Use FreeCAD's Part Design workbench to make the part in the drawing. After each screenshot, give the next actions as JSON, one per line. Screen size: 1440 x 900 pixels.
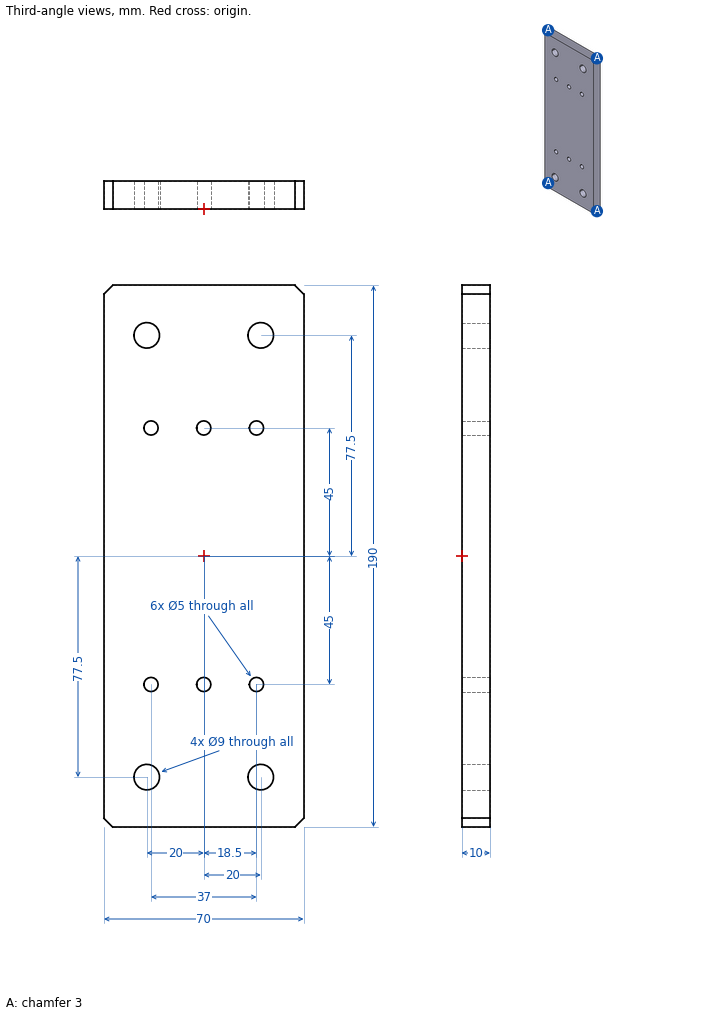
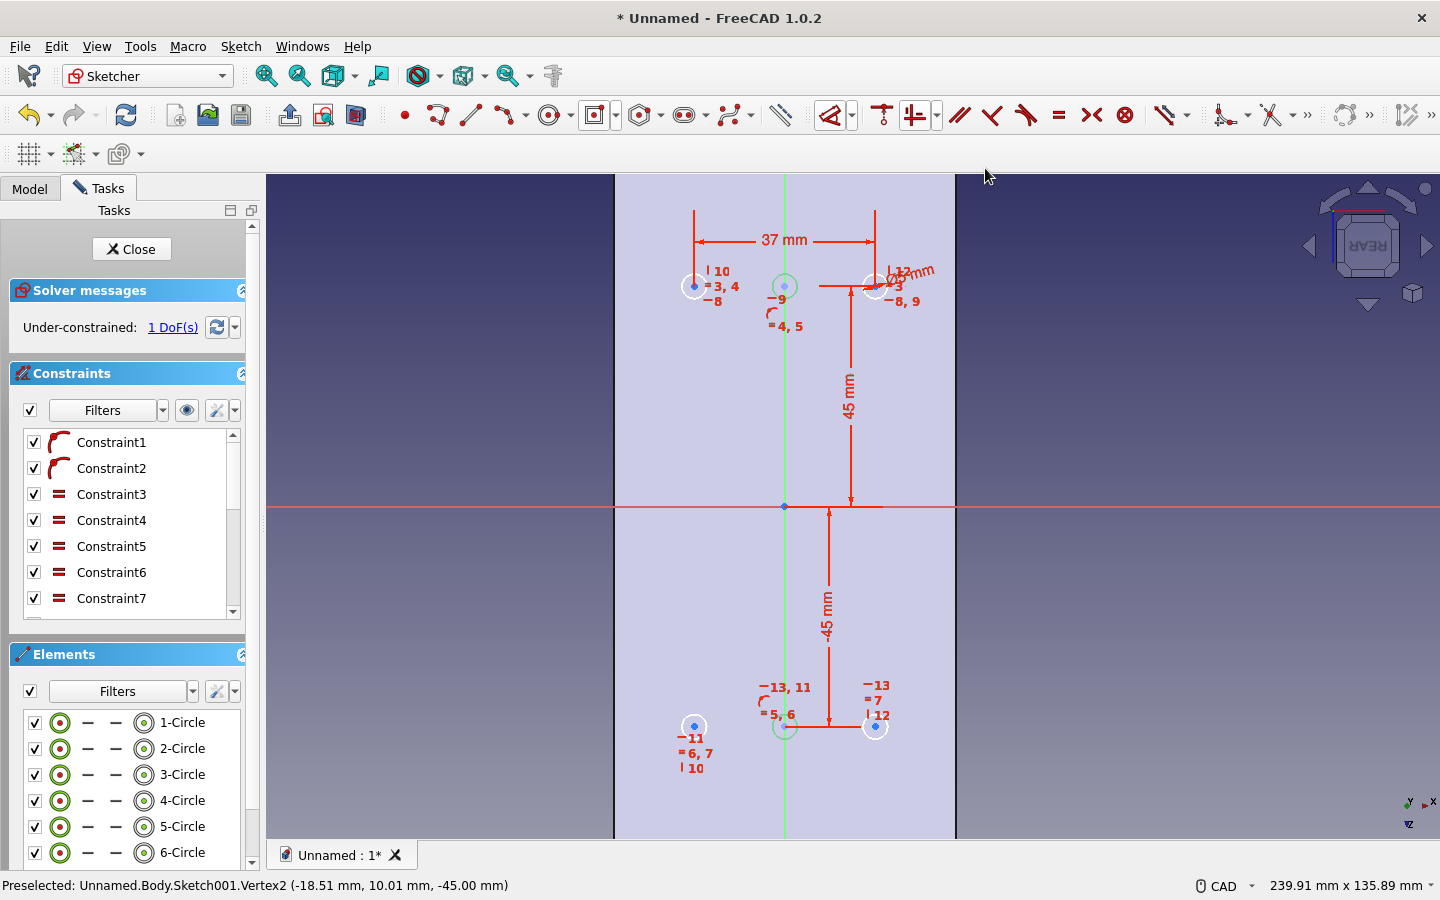
{"action": "left_click", "coordinate": [875, 286]}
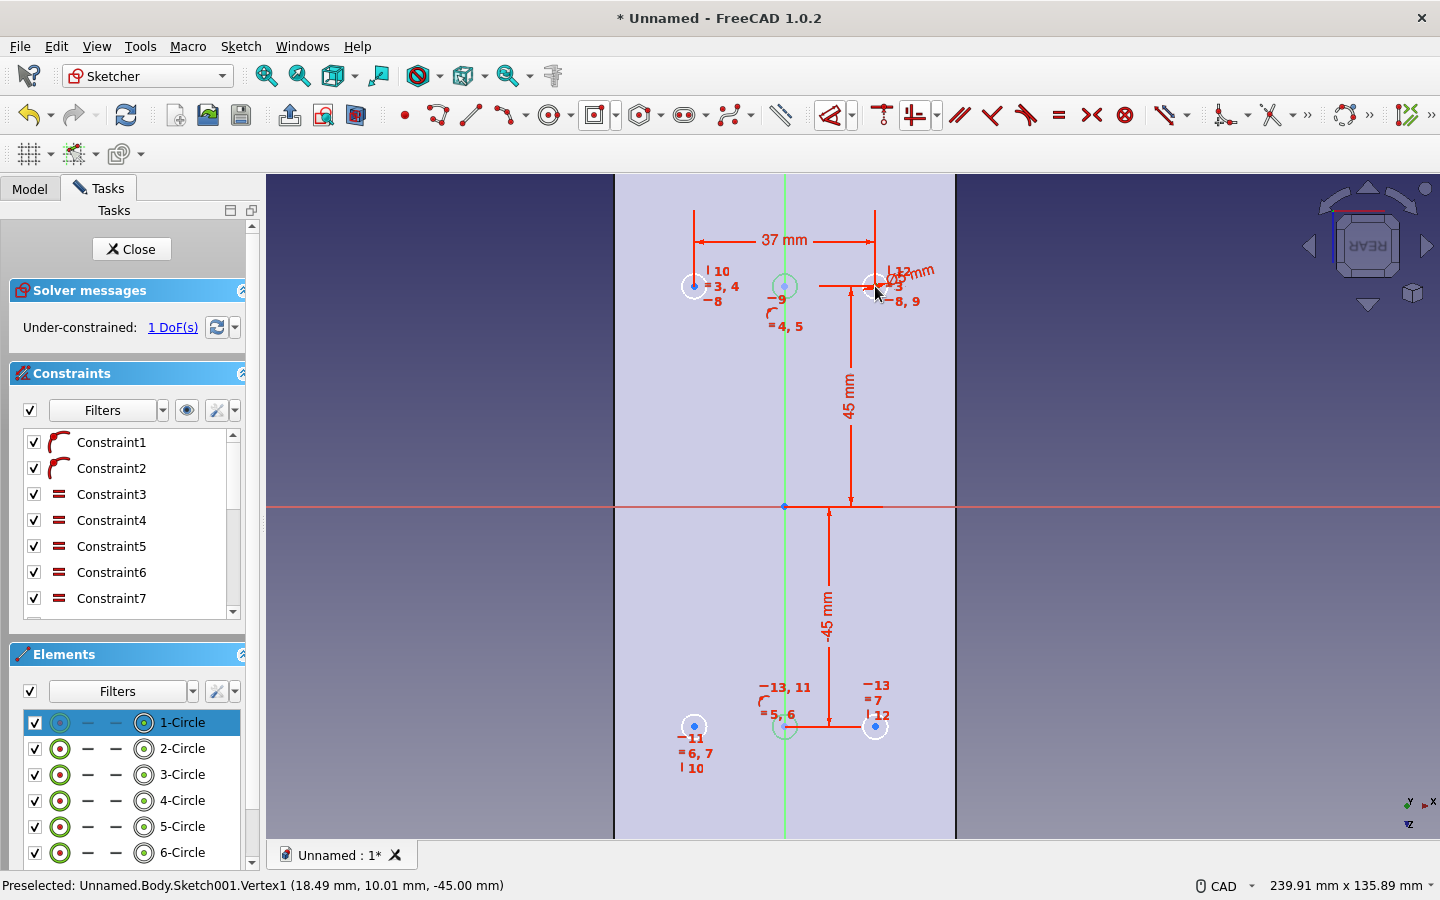
{"action": "left_click", "coordinate": [852, 116]}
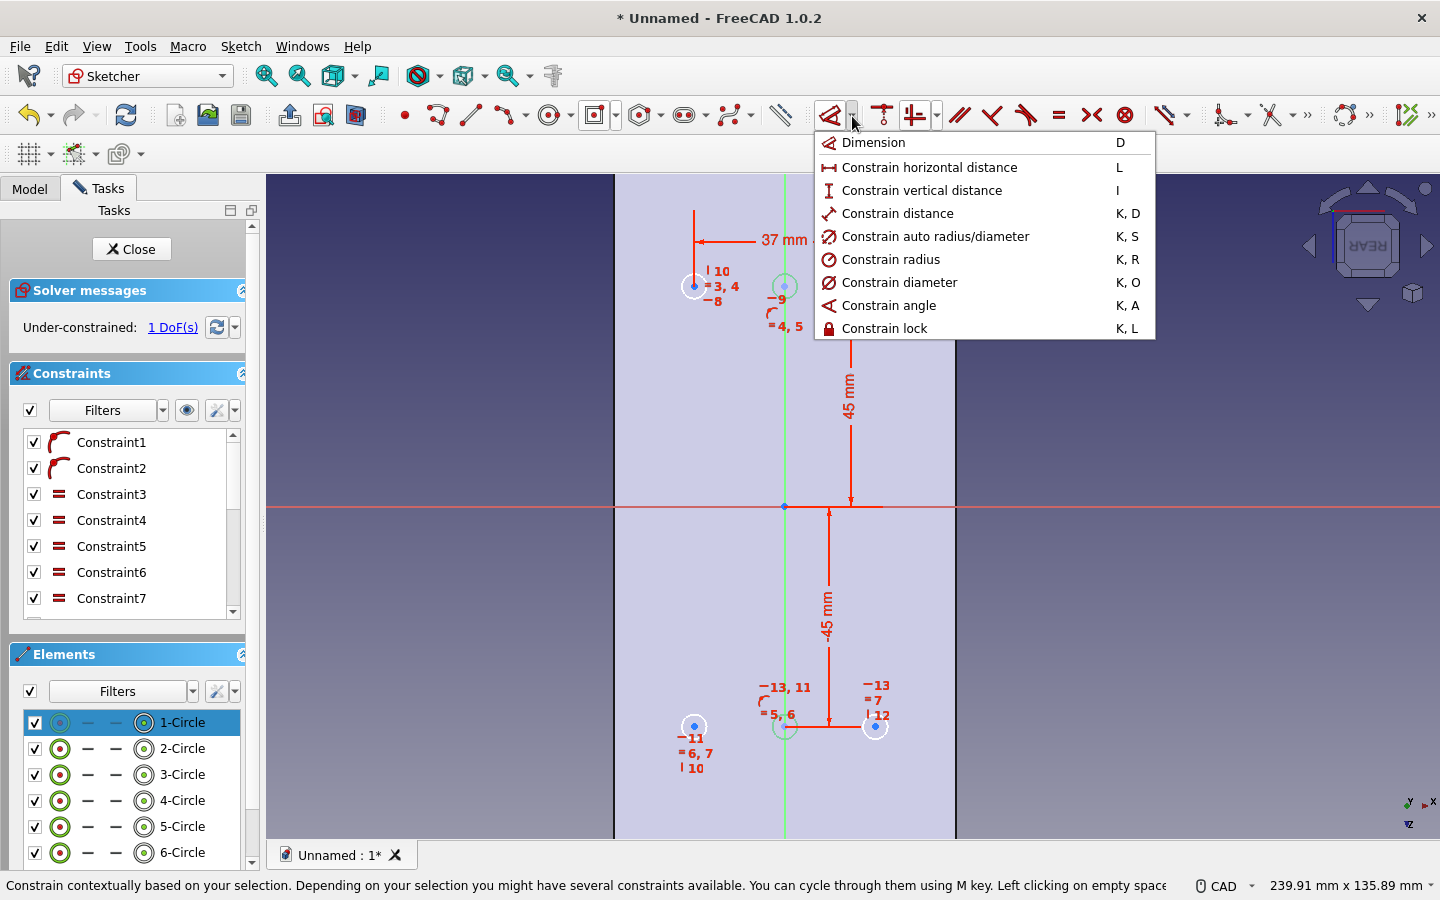
{"action": "left_click", "coordinate": [985, 168]}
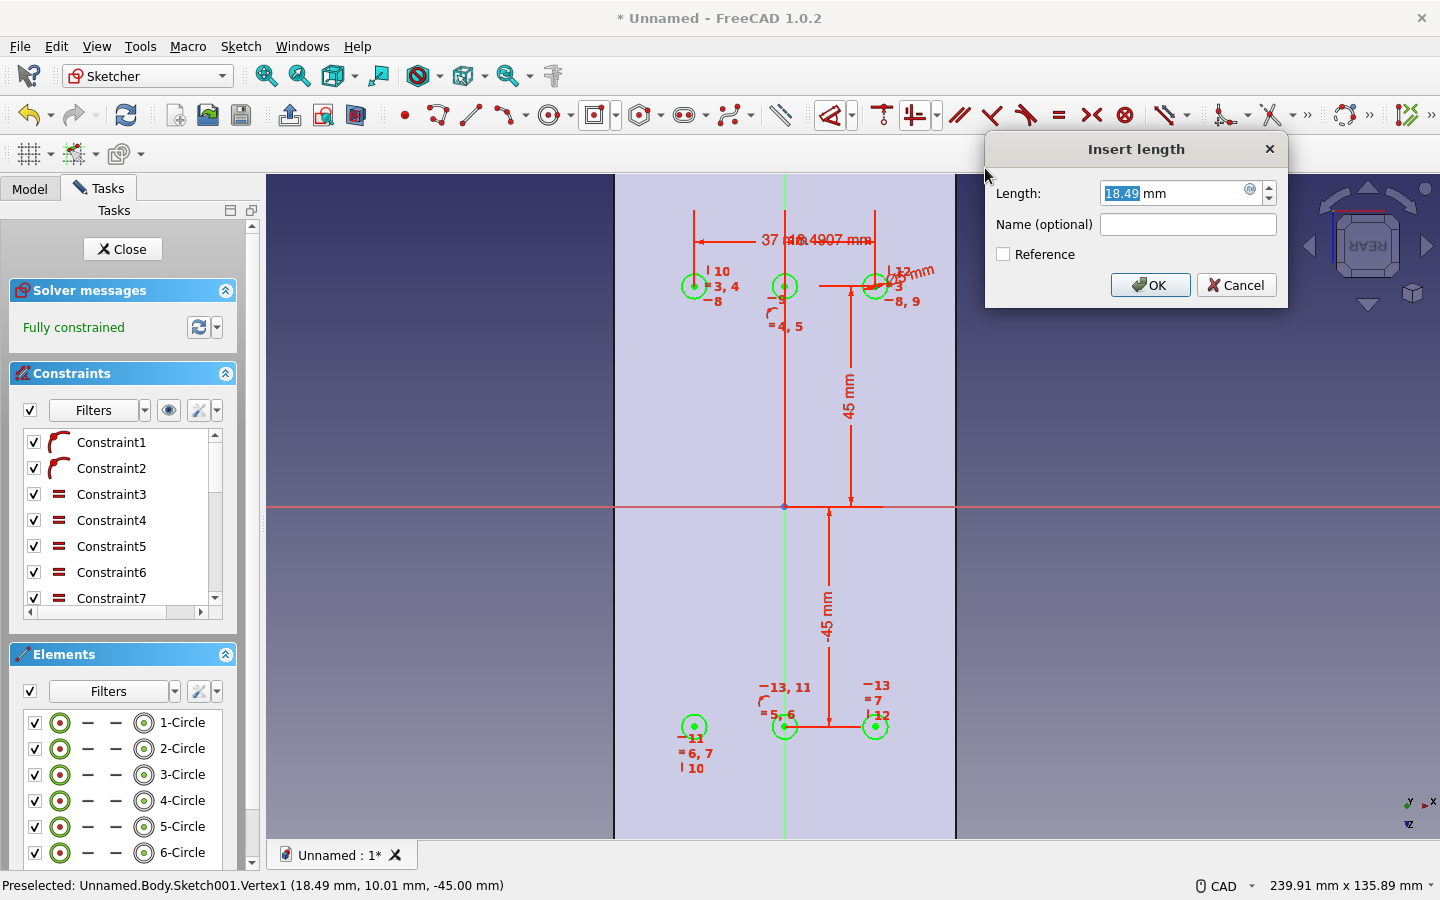
{"action": "type", "text": "18.5"}
{"action": "key", "text": "Return"}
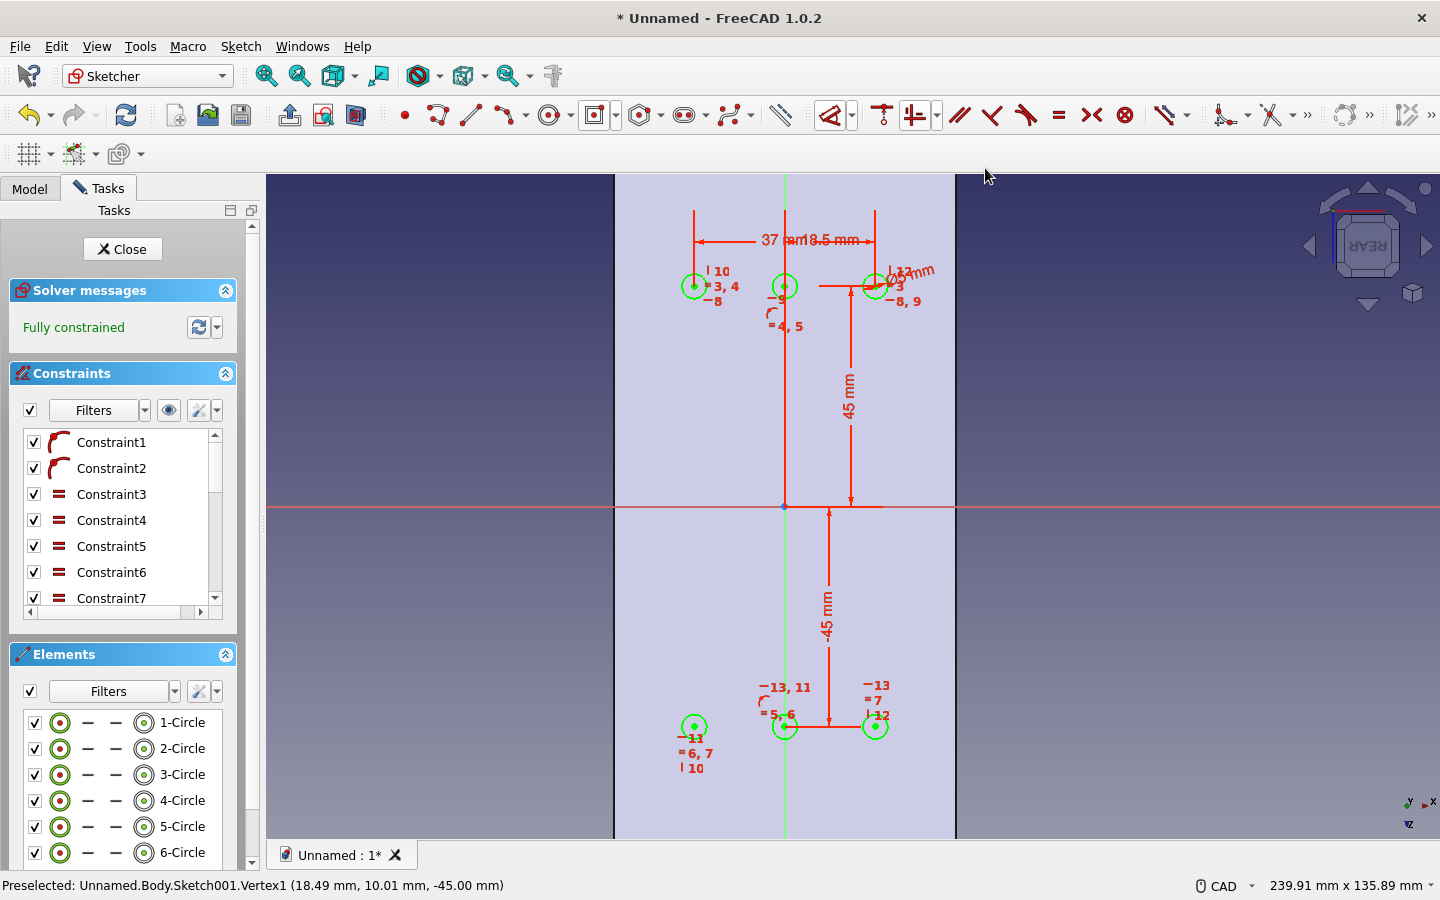
{"action": "left_click", "coordinate": [123, 249]}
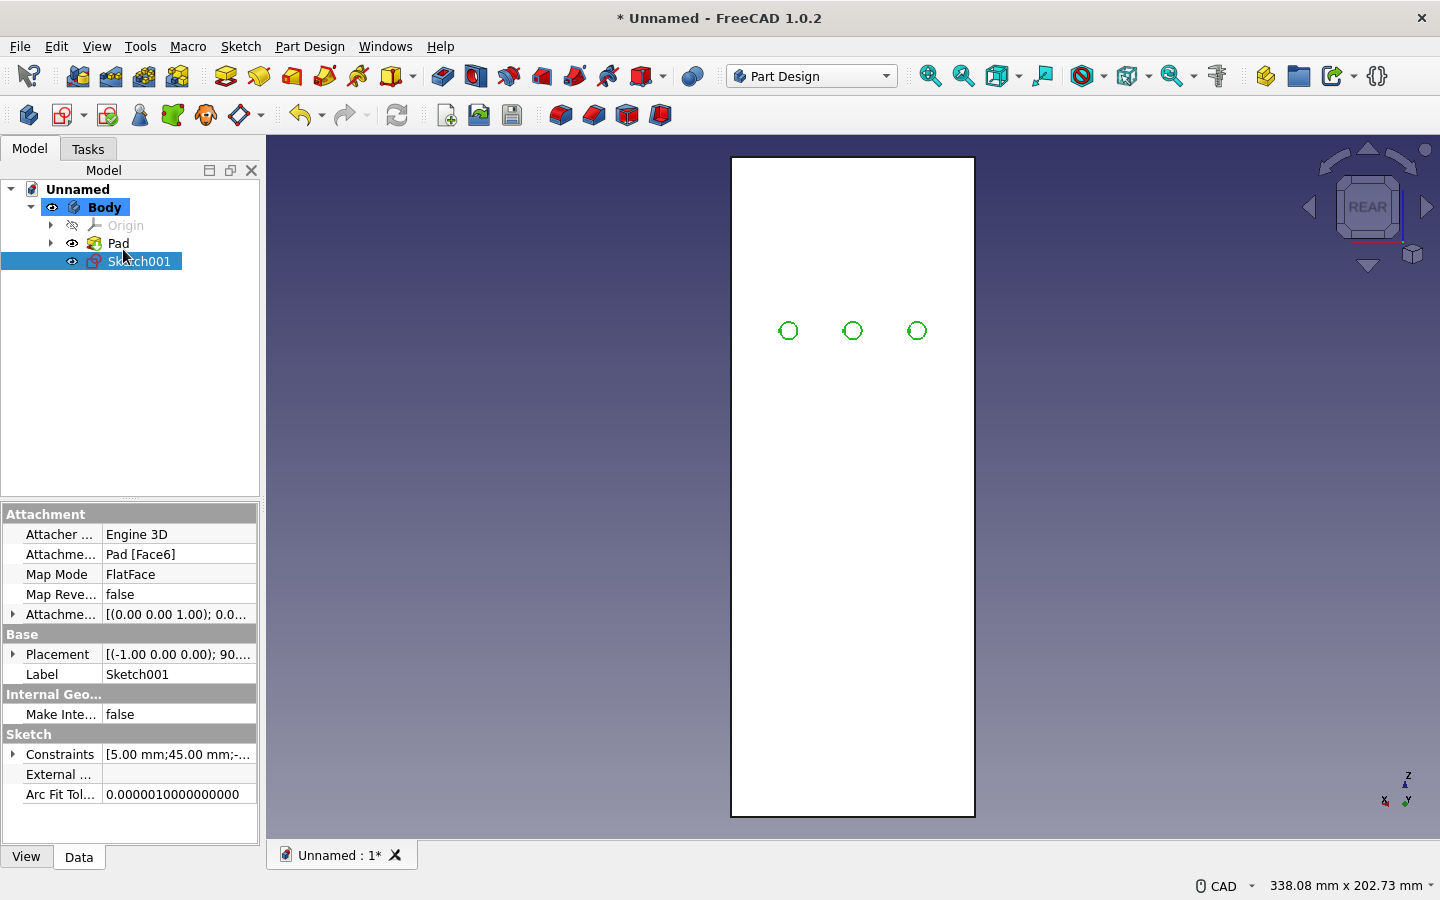
{"action": "left_click", "coordinate": [476, 76]}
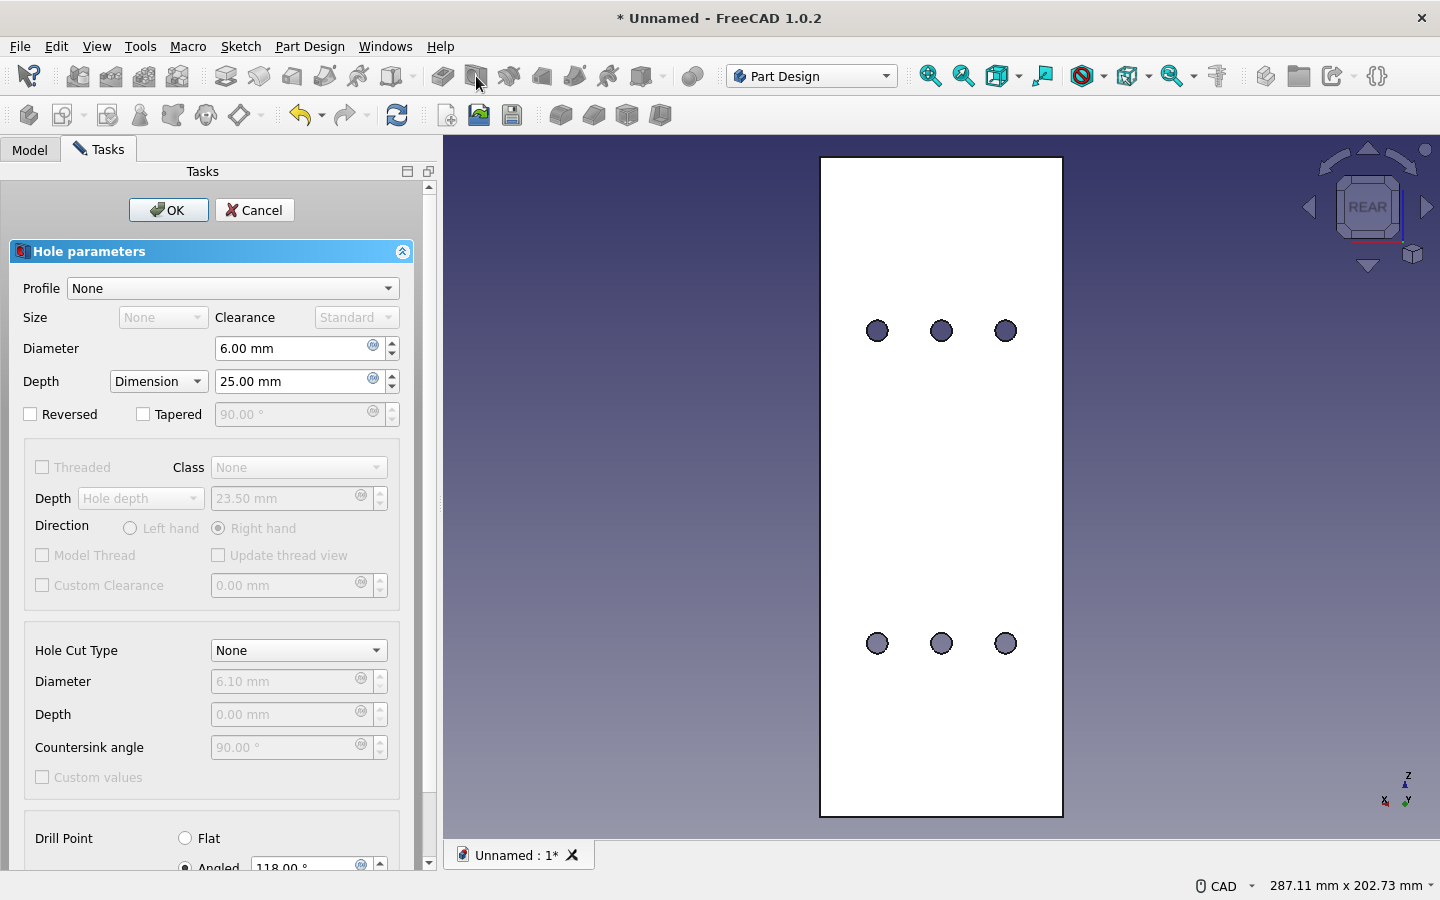
{"action": "triple_click", "coordinate": [300, 348]}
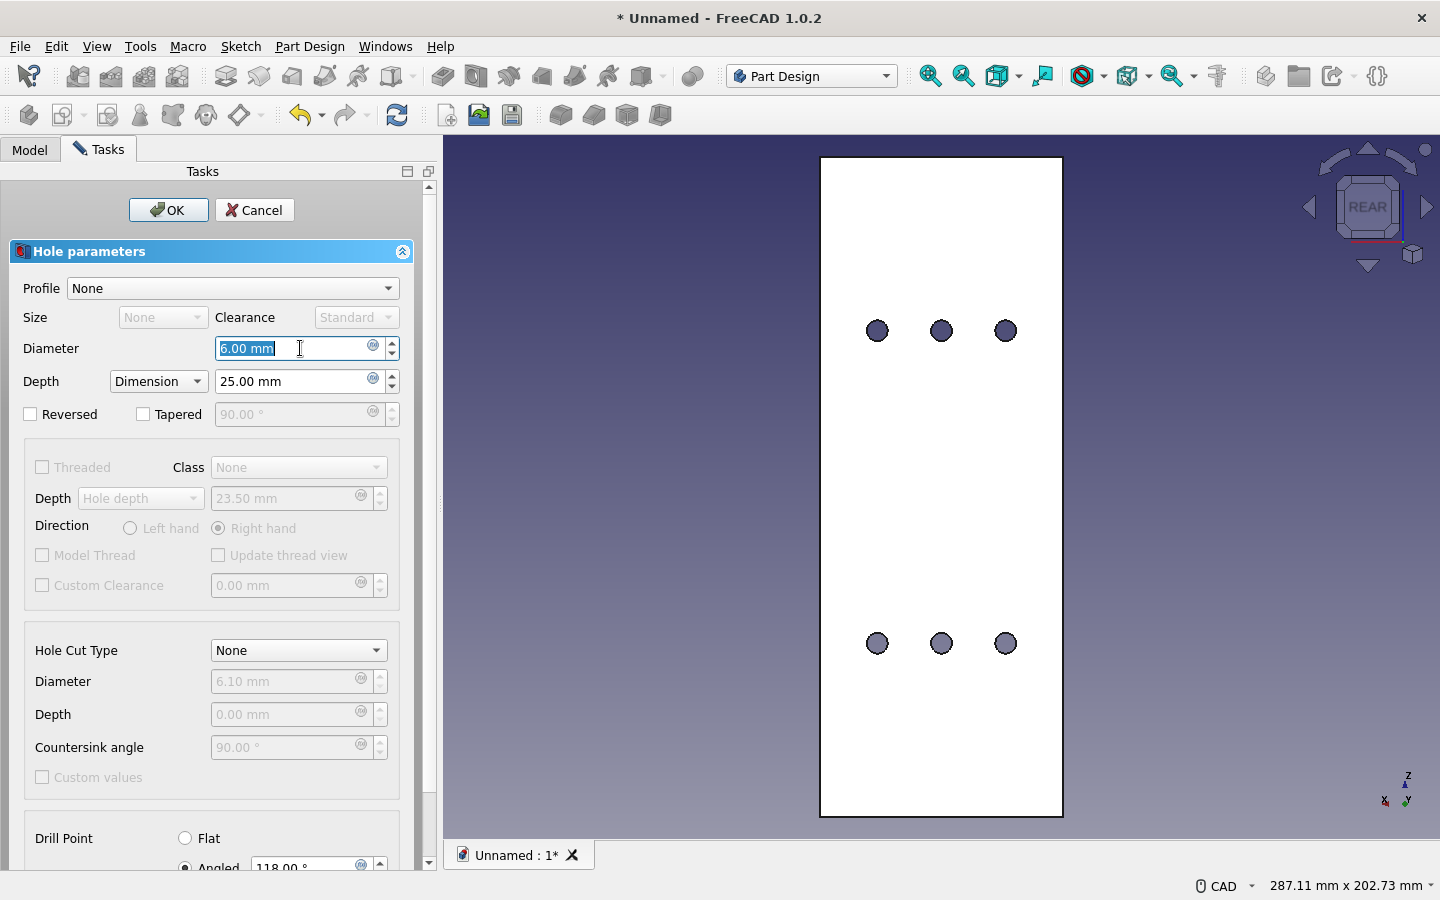
{"action": "type", "text": "5"}
{"action": "key", "text": "Tab"}